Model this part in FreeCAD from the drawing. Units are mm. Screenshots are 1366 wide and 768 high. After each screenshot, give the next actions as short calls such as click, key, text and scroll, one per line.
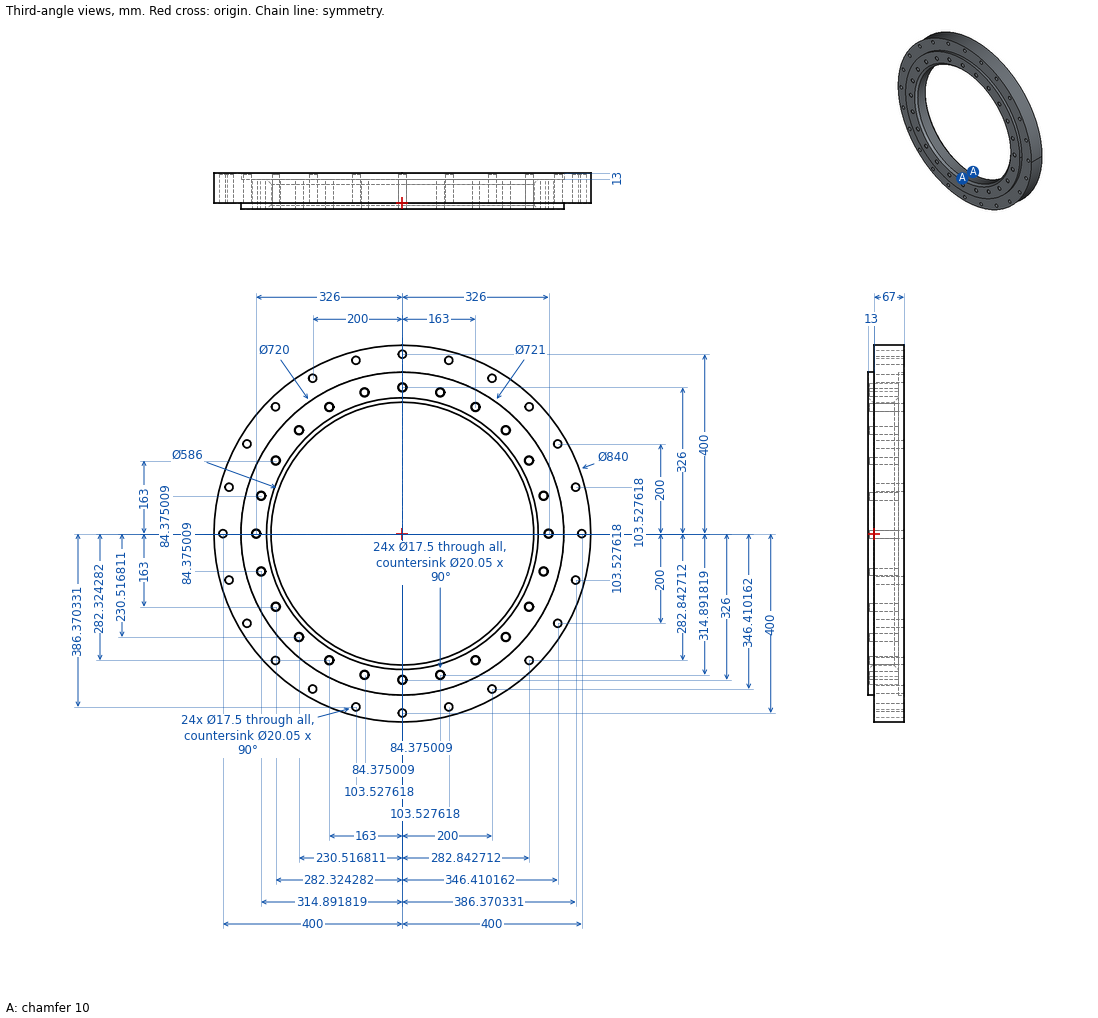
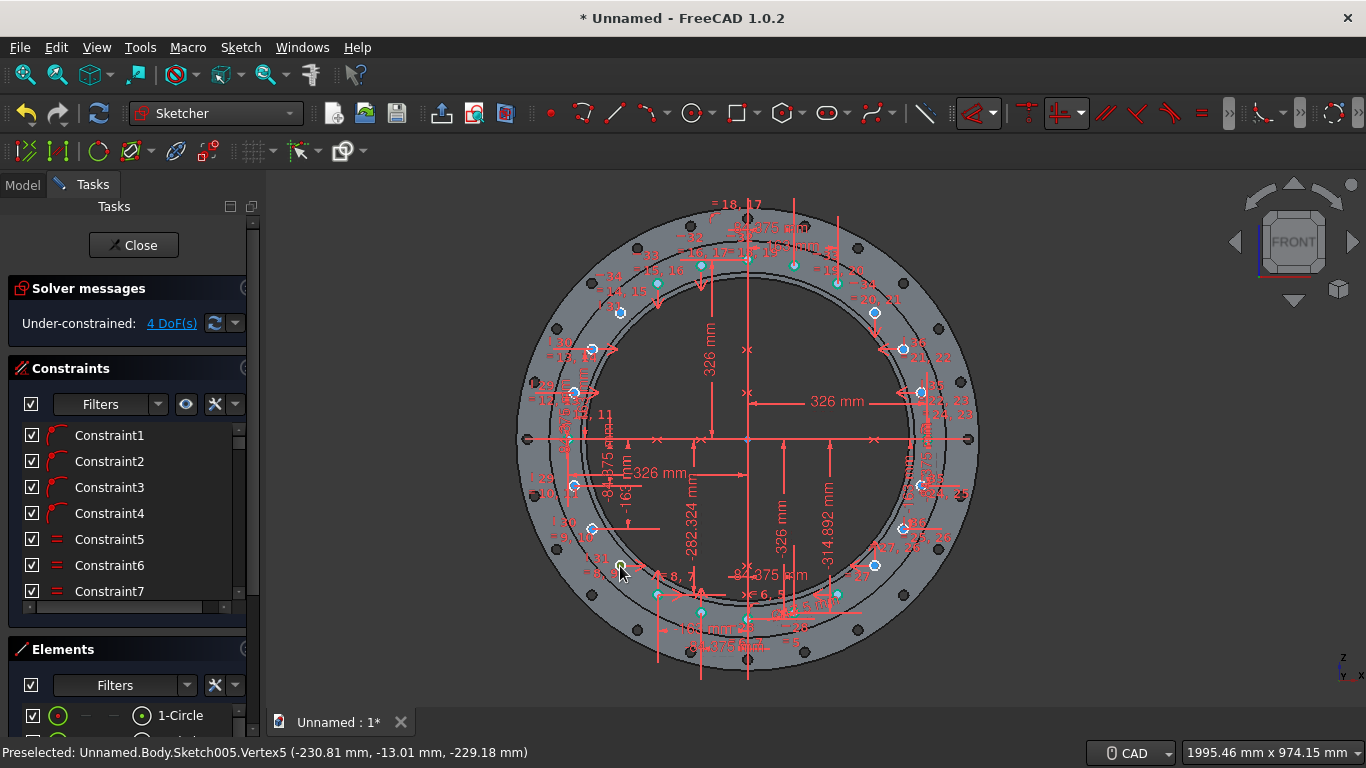
key(l)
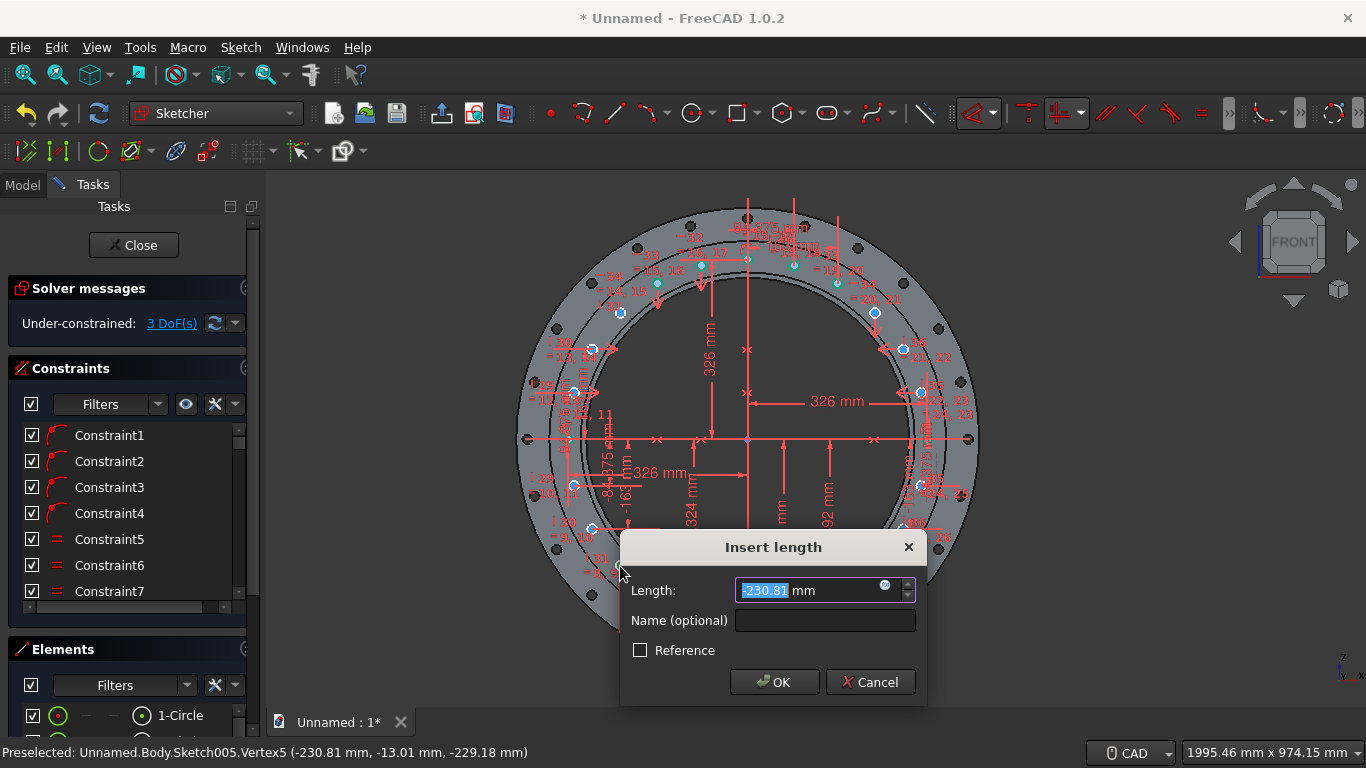
text(-230.516811)
key(Return)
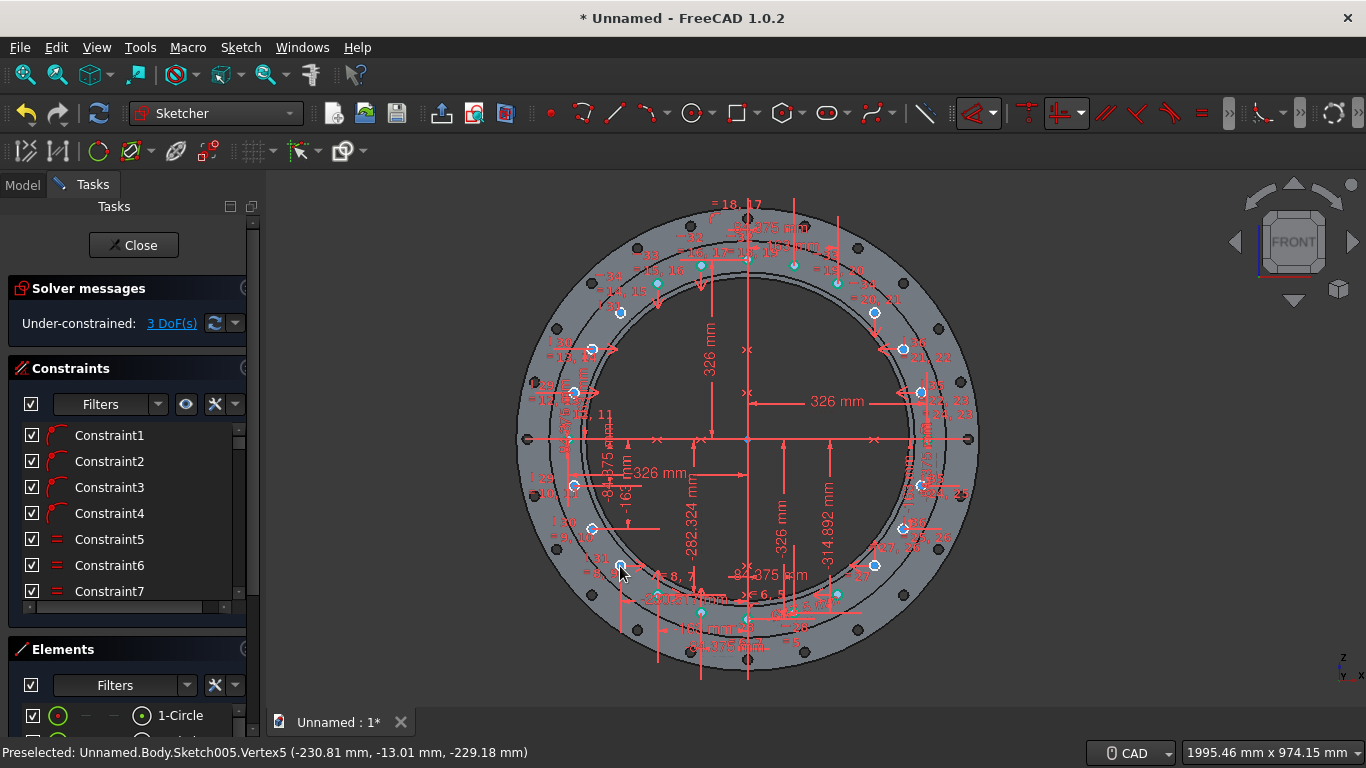
click(621, 566)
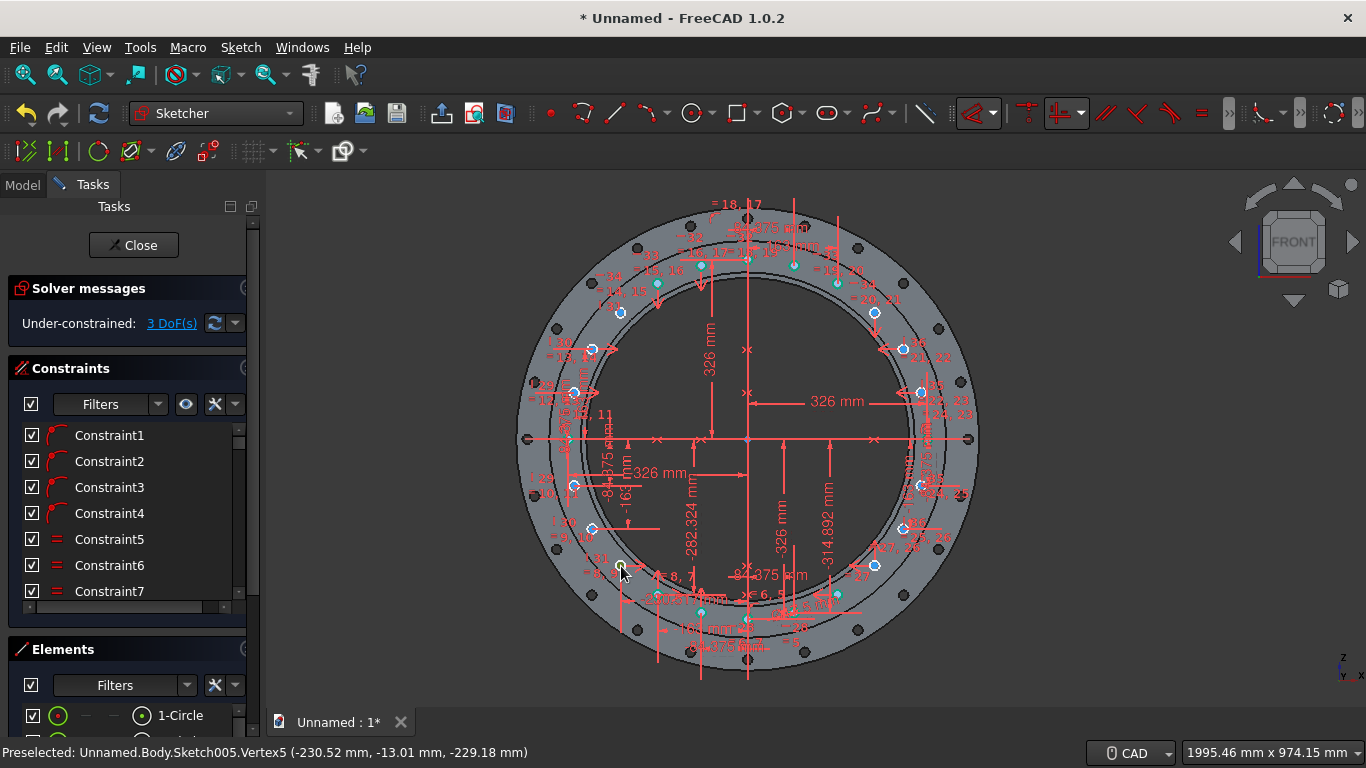
click(996, 114)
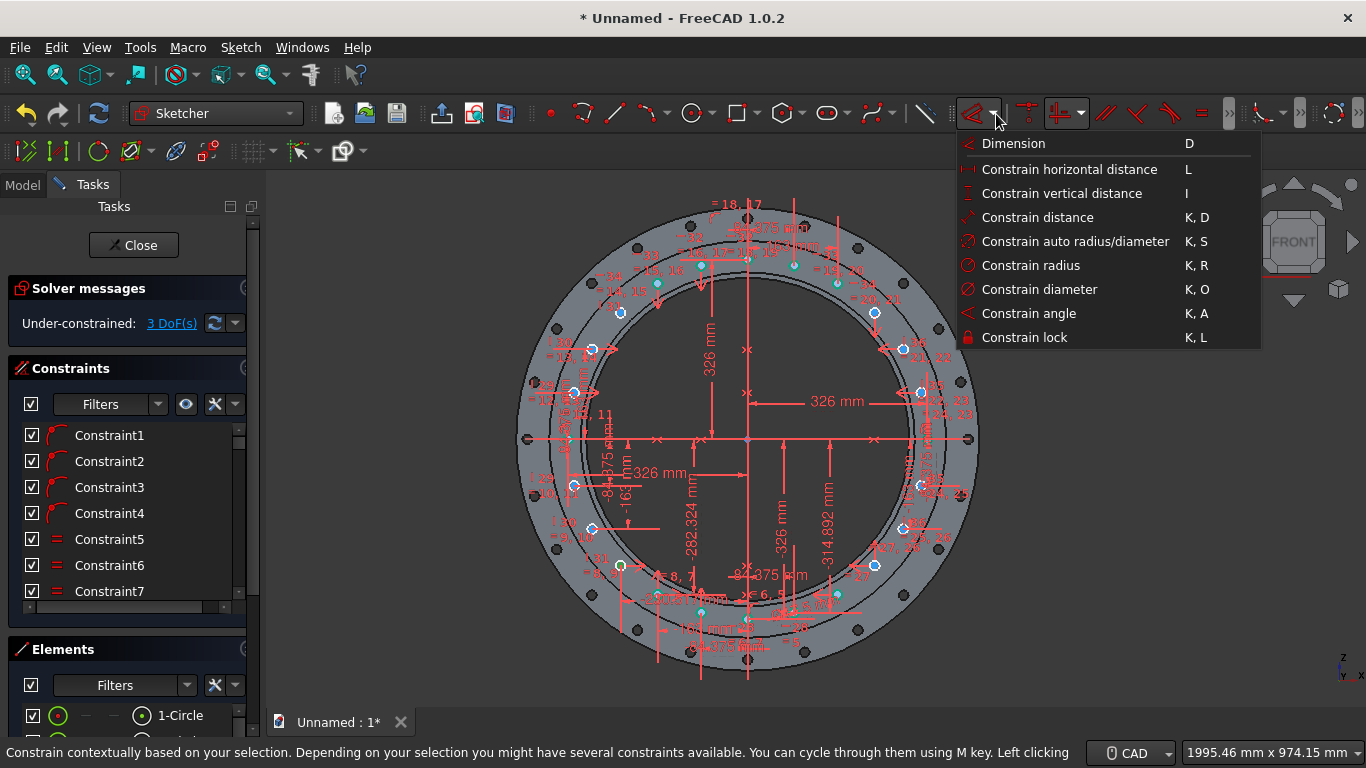
click(1109, 193)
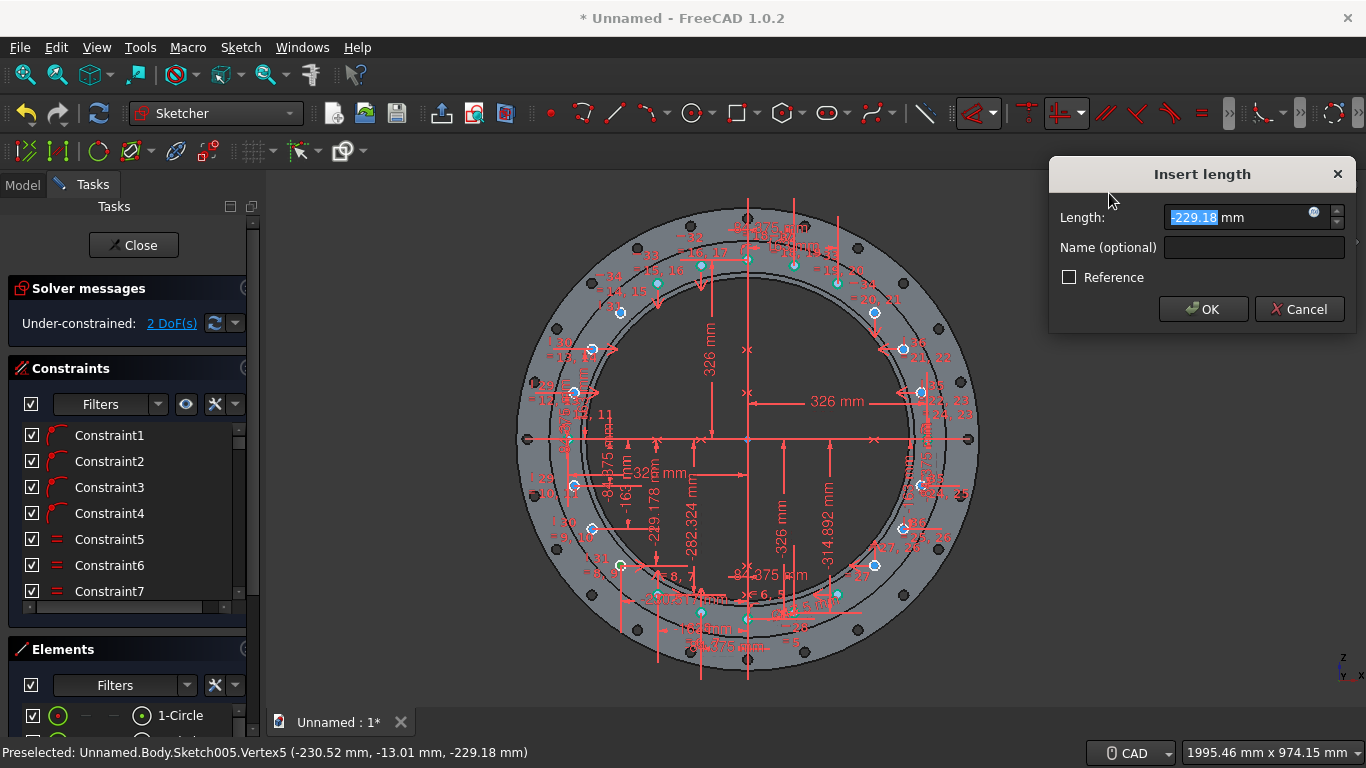
text(-230.516811)
key(Return)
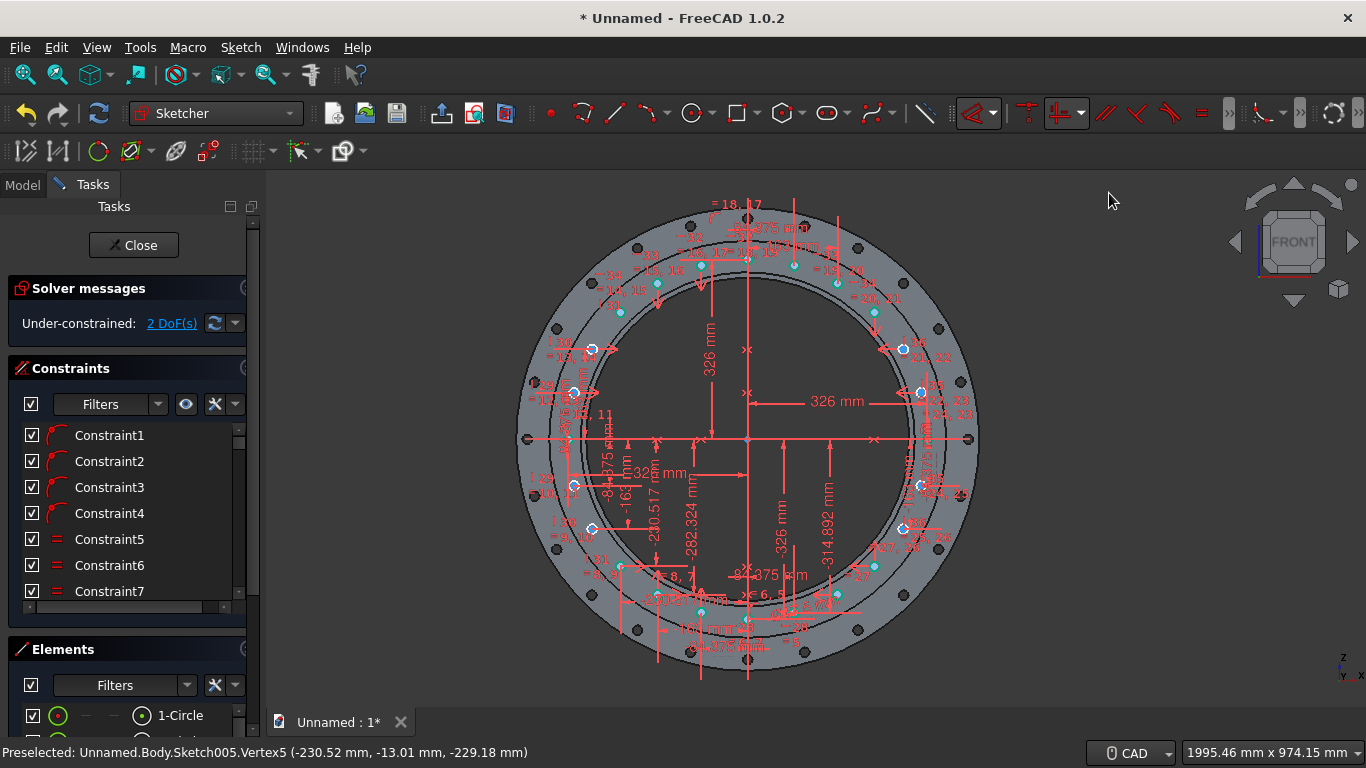
click(592, 529)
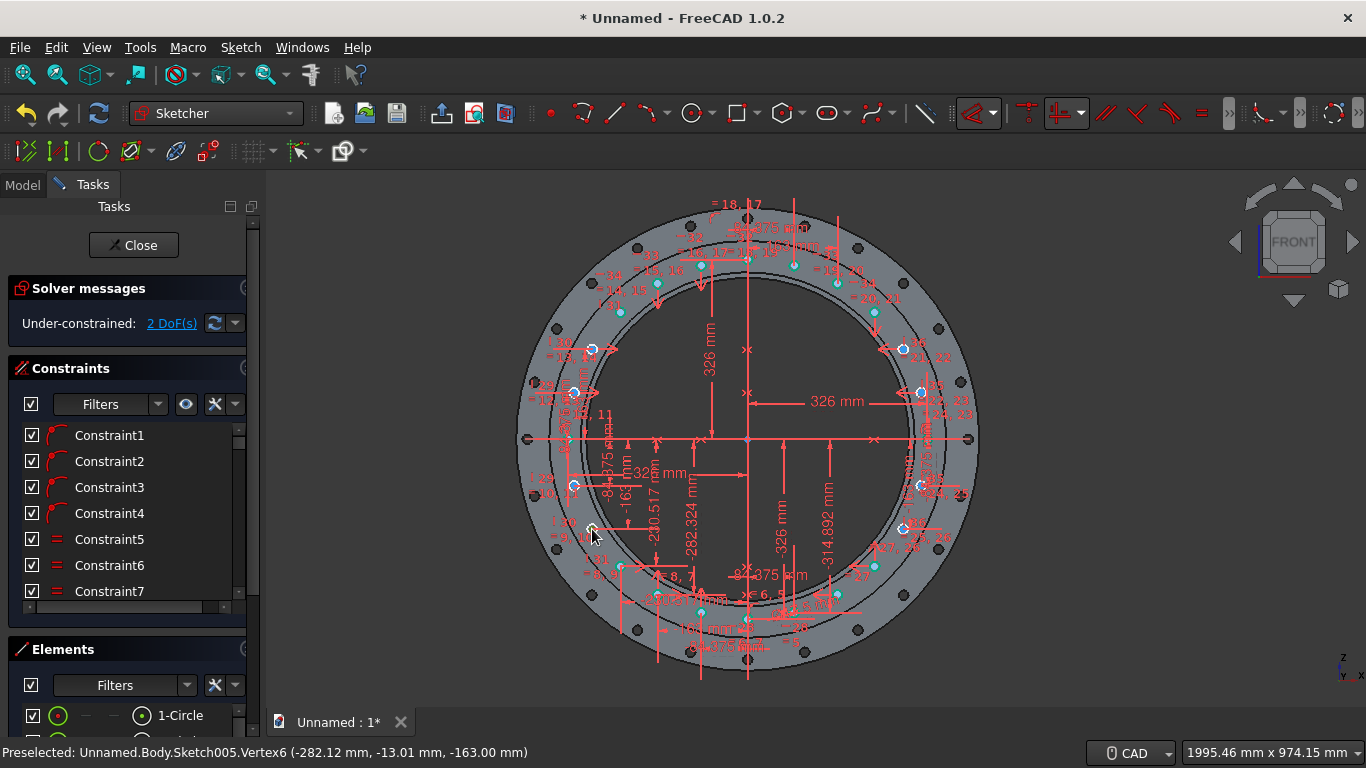
key(l)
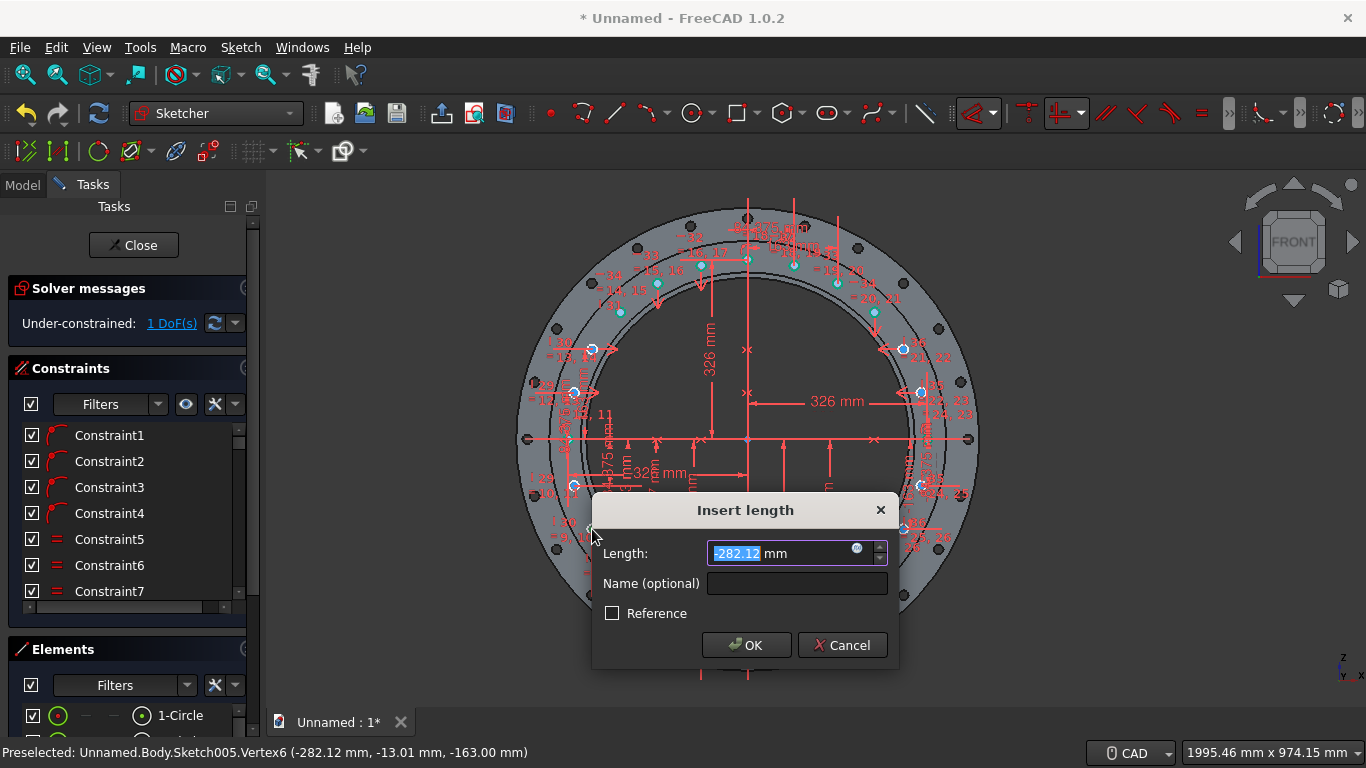
text(-282.324282)
key(Return)